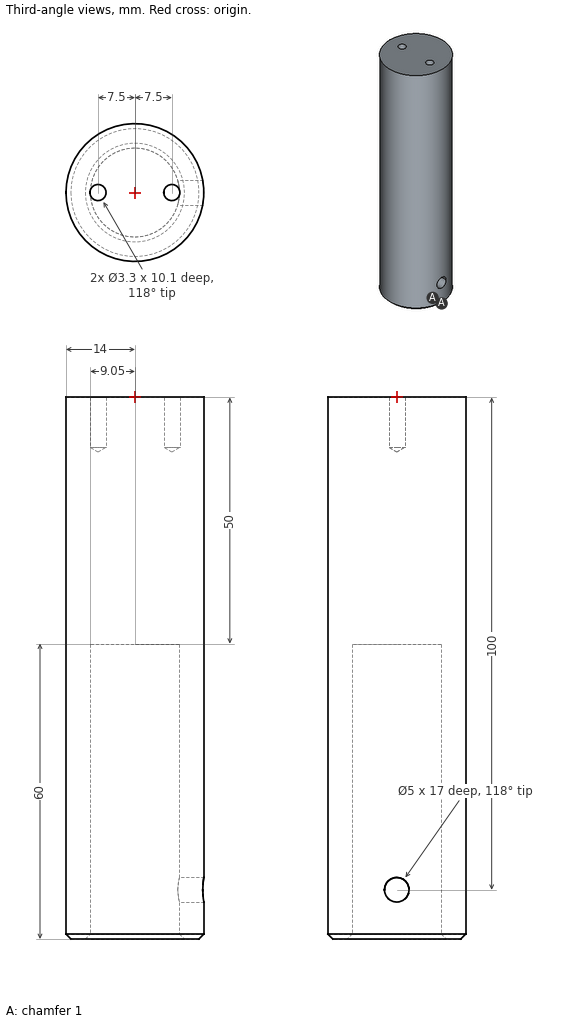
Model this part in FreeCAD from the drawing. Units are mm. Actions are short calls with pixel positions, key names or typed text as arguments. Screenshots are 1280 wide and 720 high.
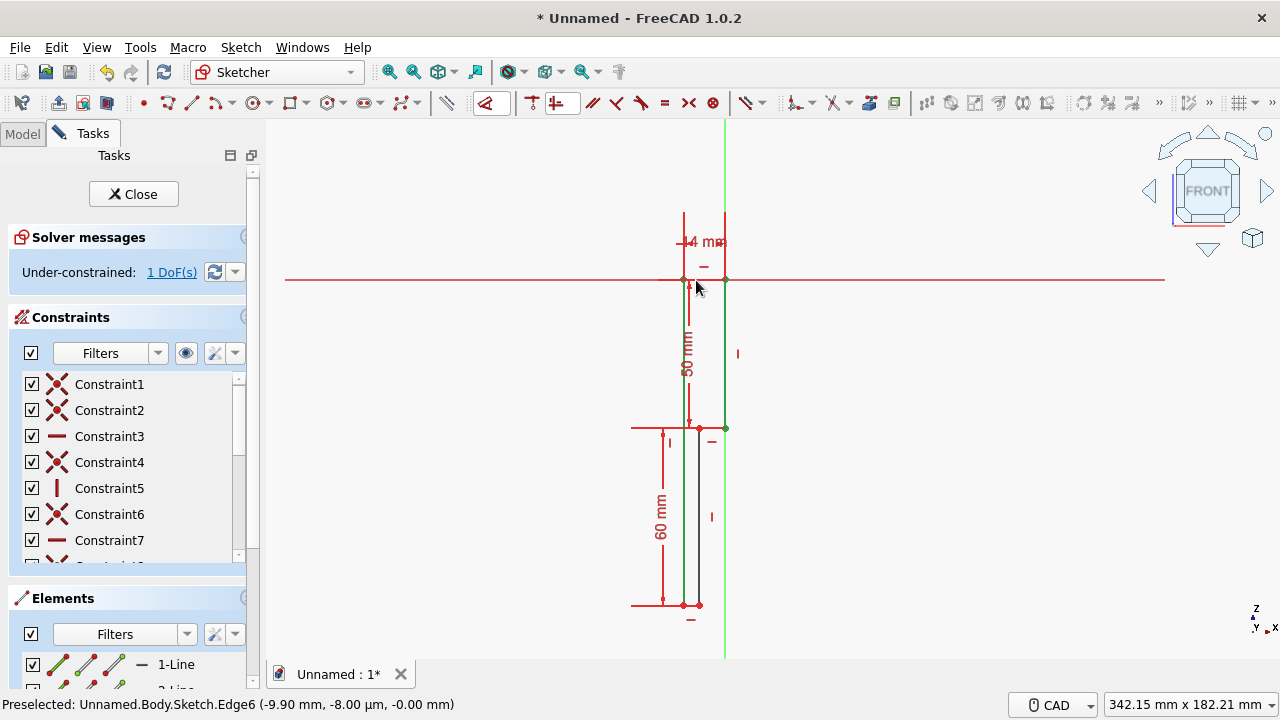
scroll(715, 428, up, 2)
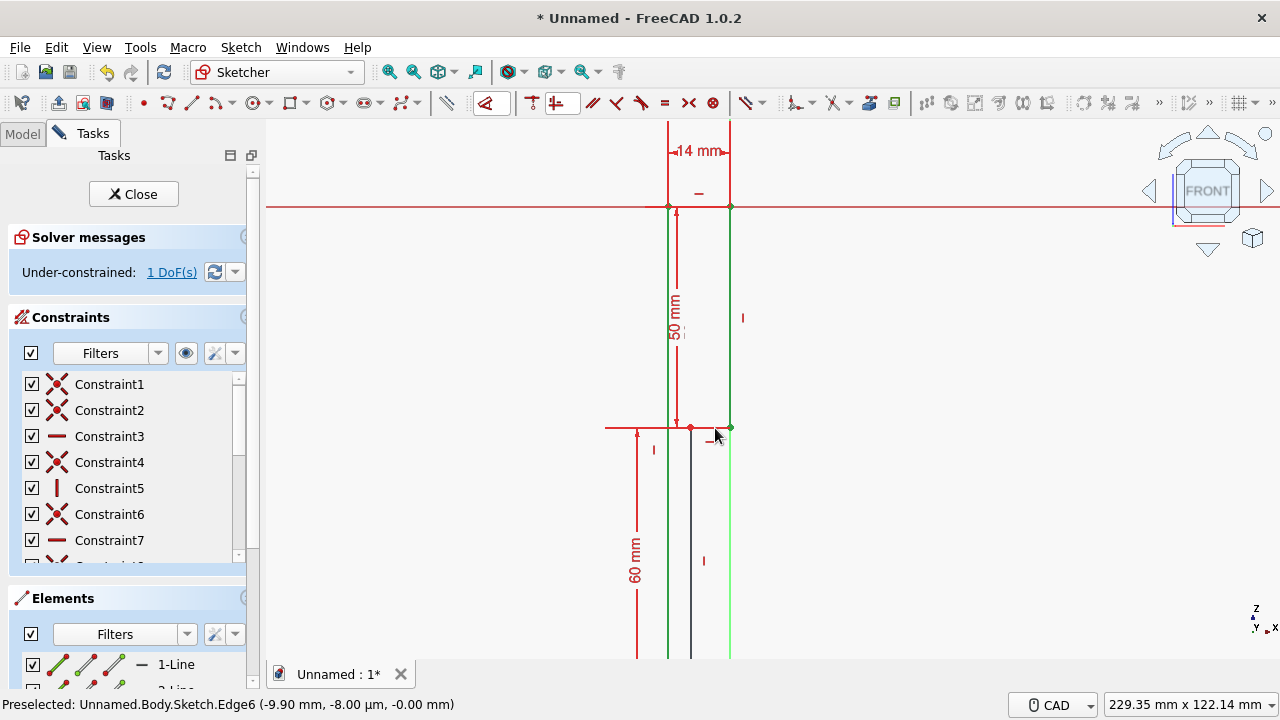
click(715, 428)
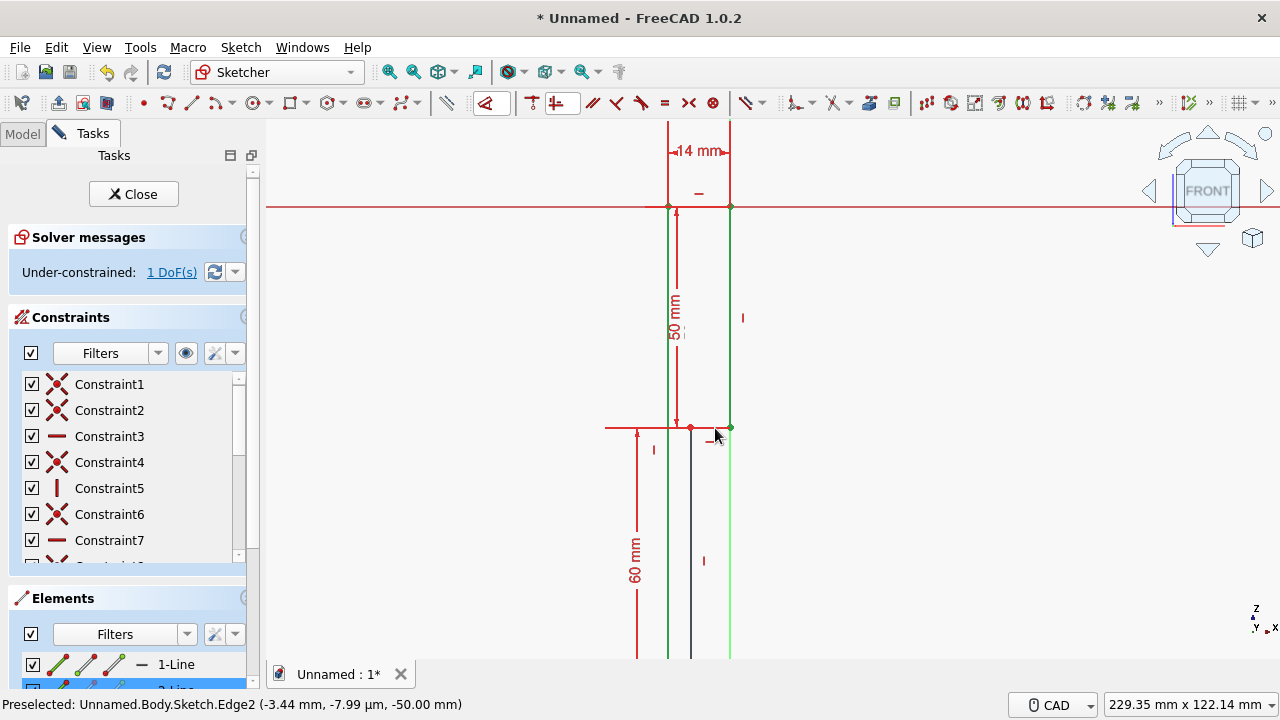
click(504, 104)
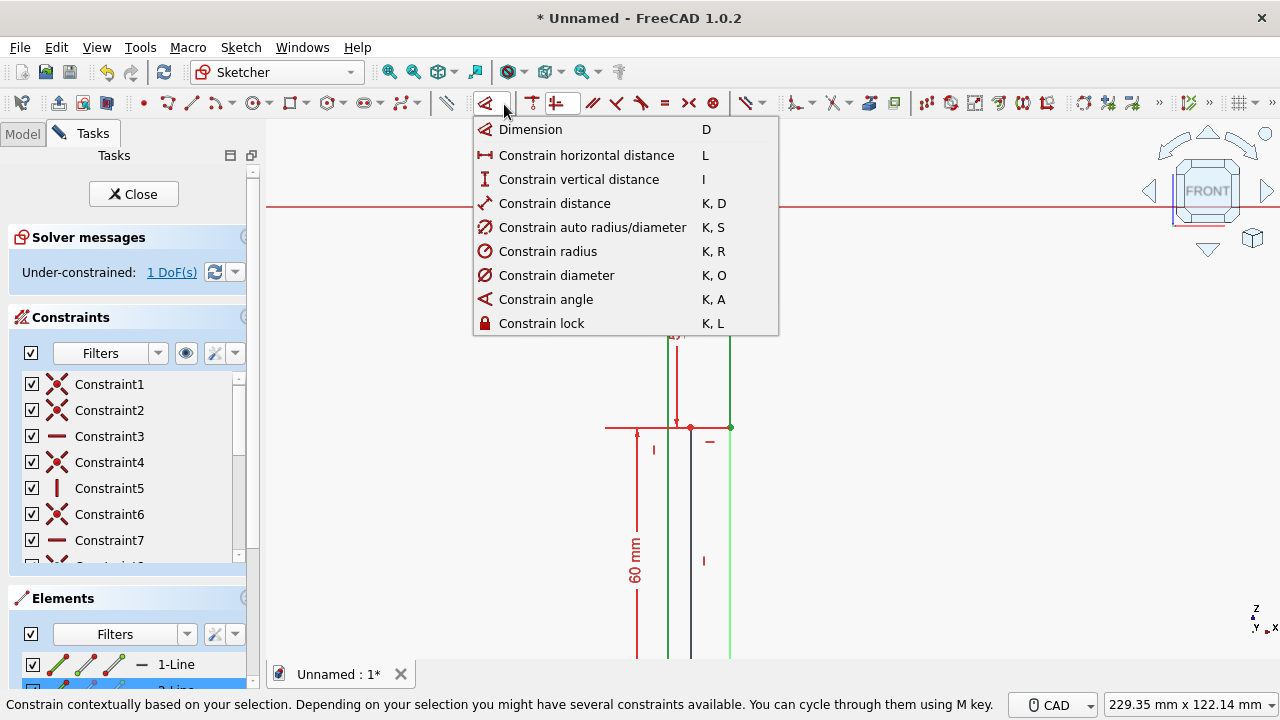
click(626, 155)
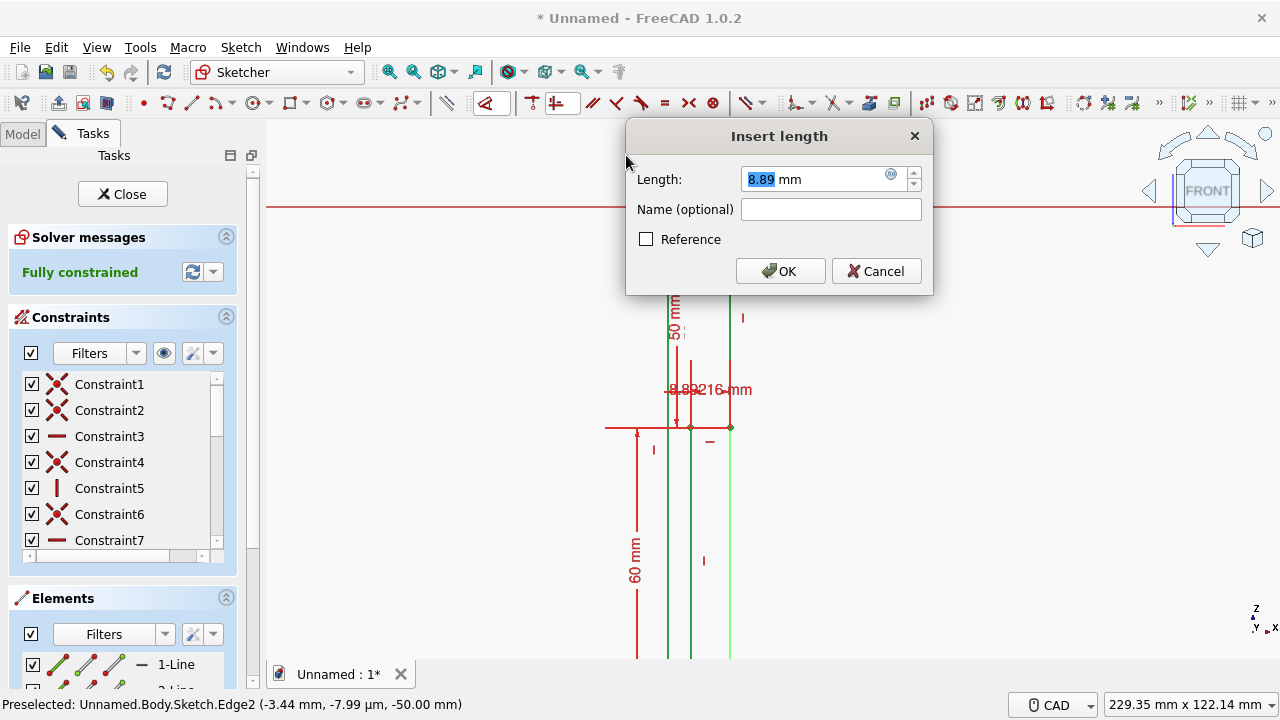
text(9.05)
key(Return)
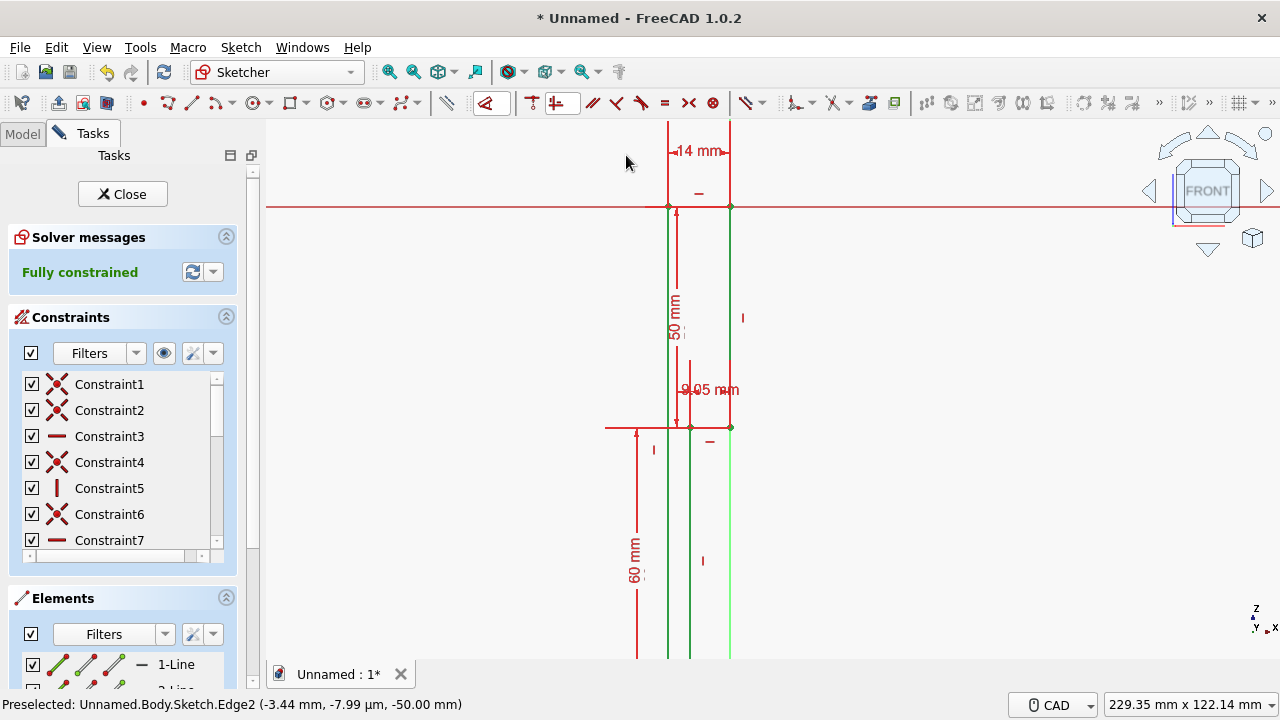
click(123, 194)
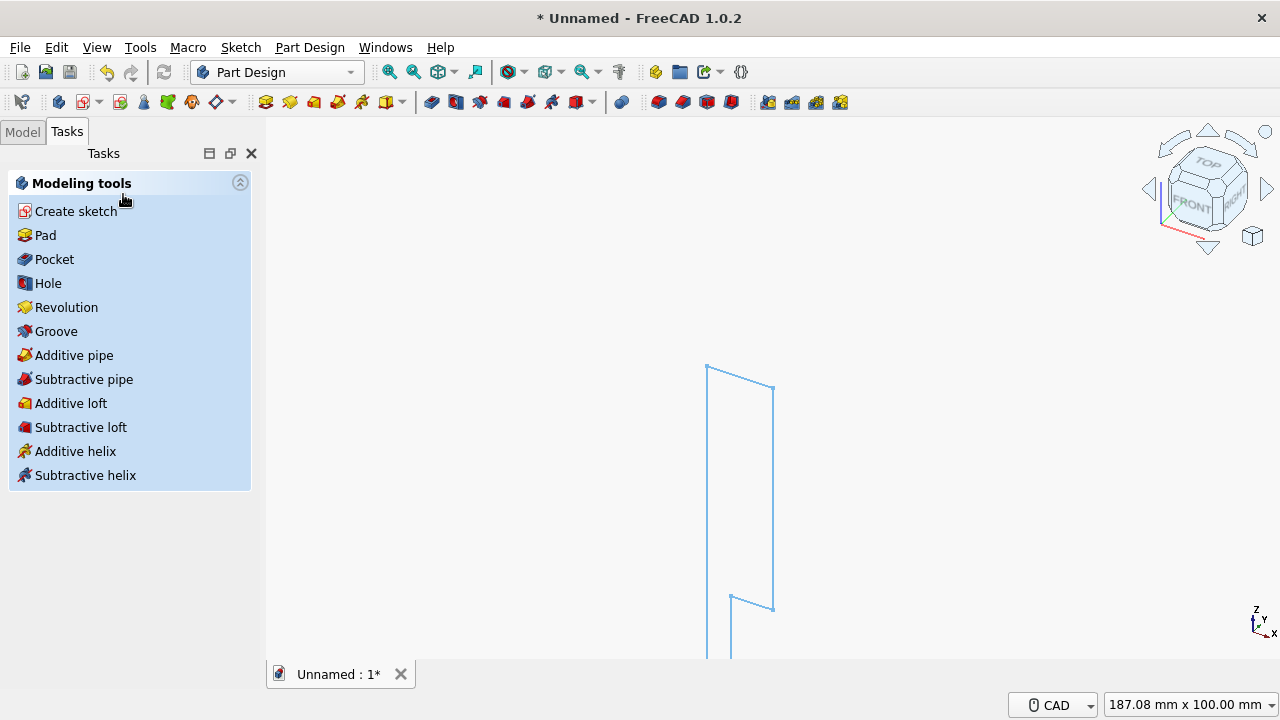
click(290, 102)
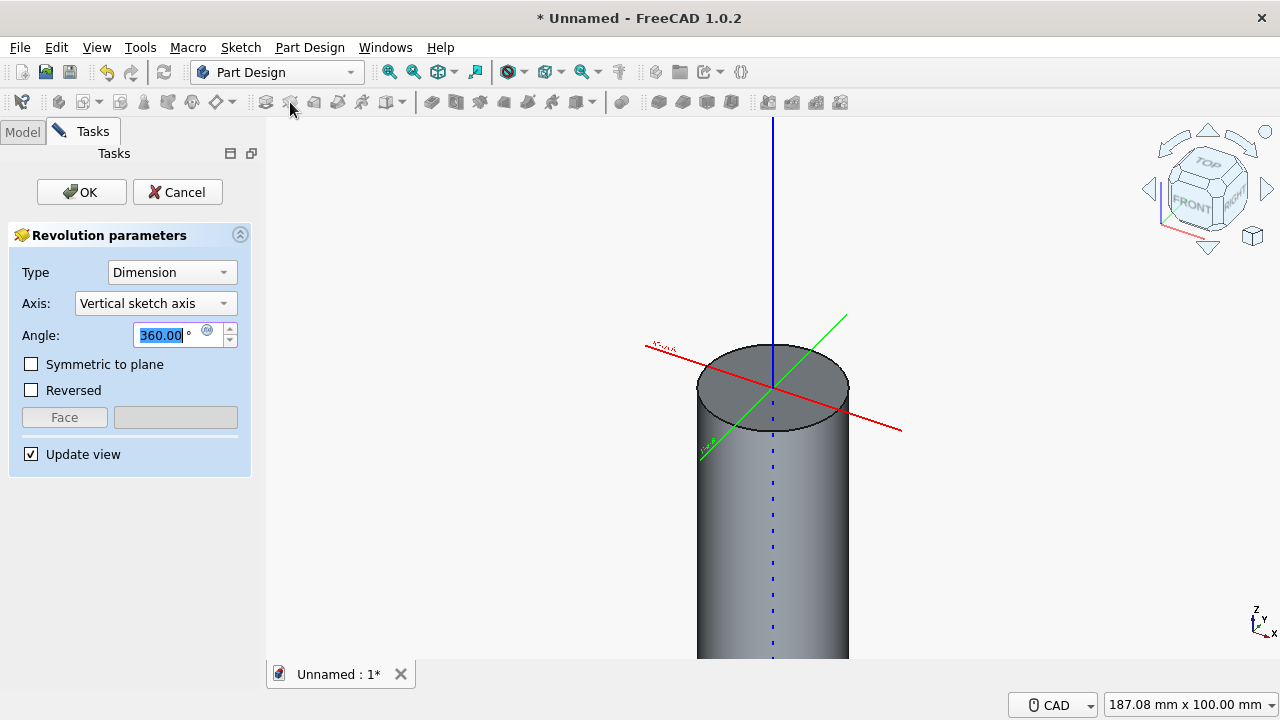
click(82, 192)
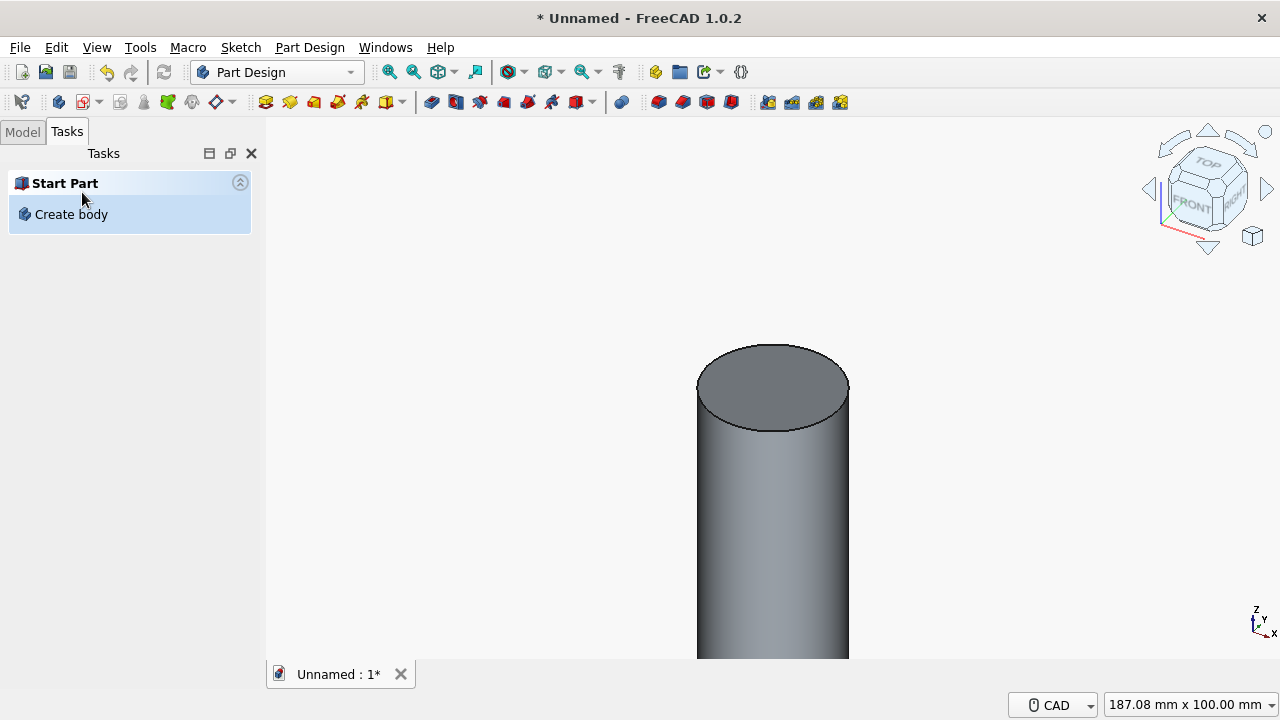
click(390, 72)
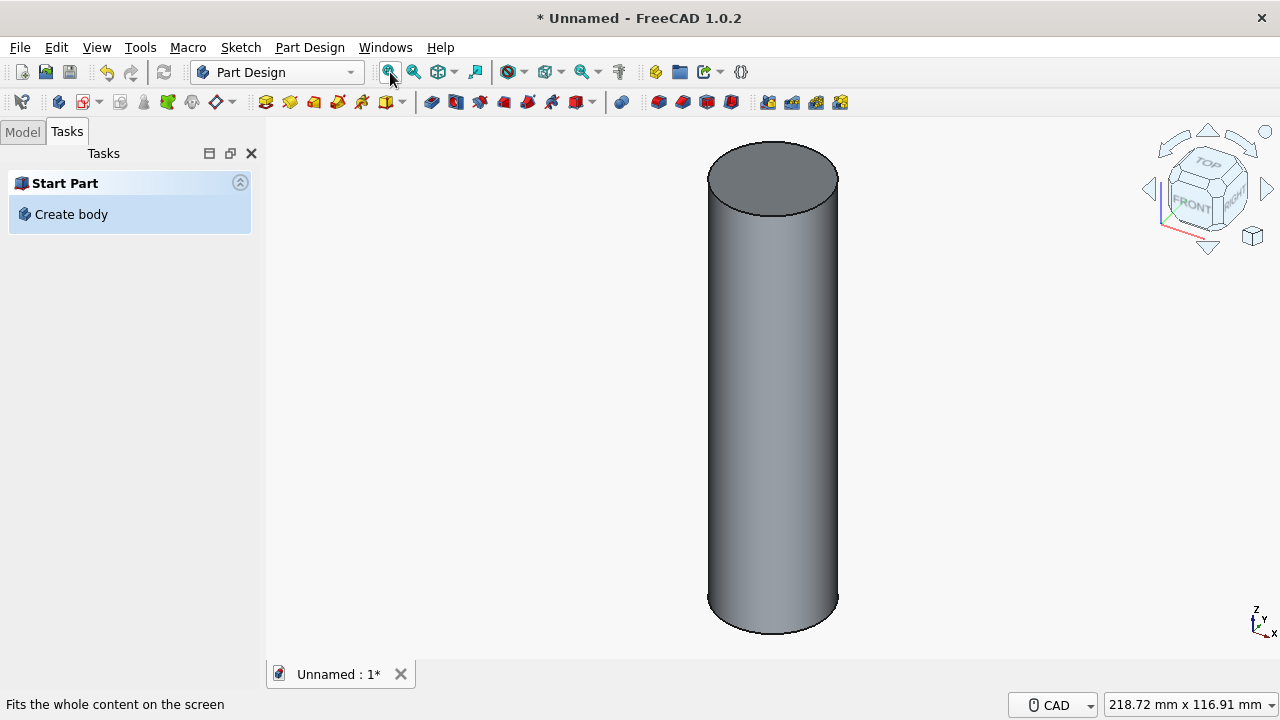
click(773, 178)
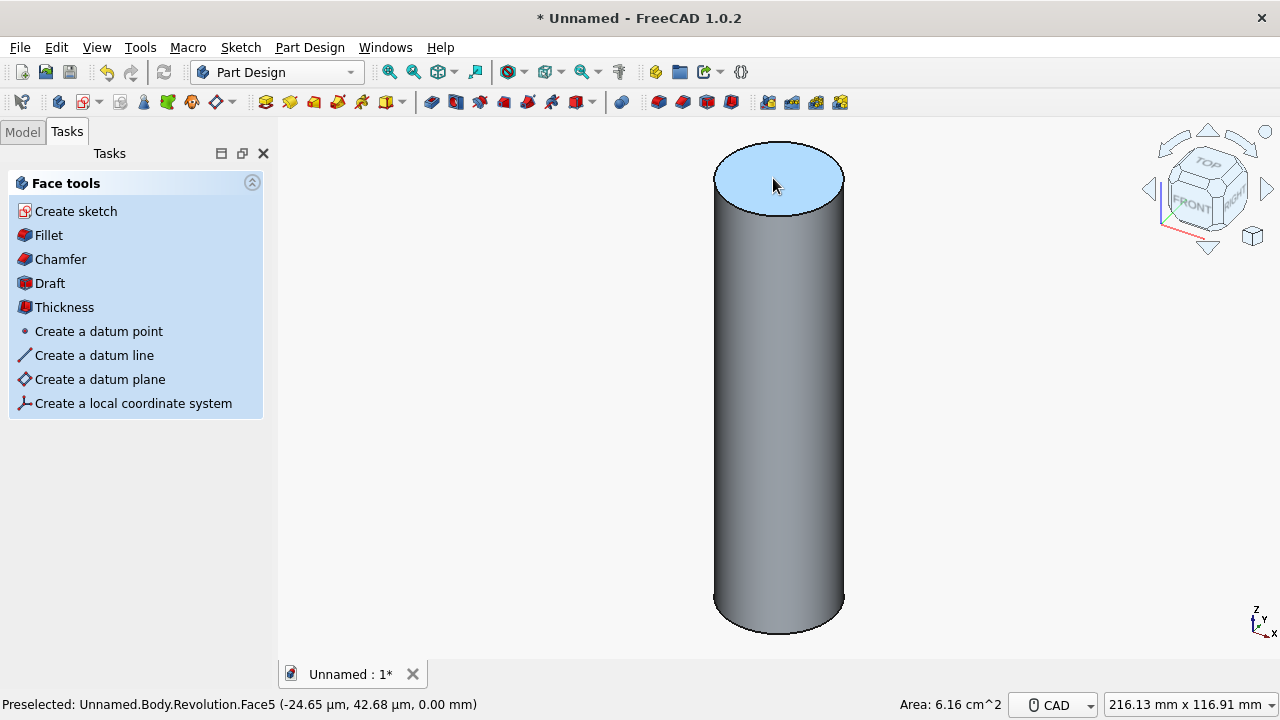
click(84, 102)